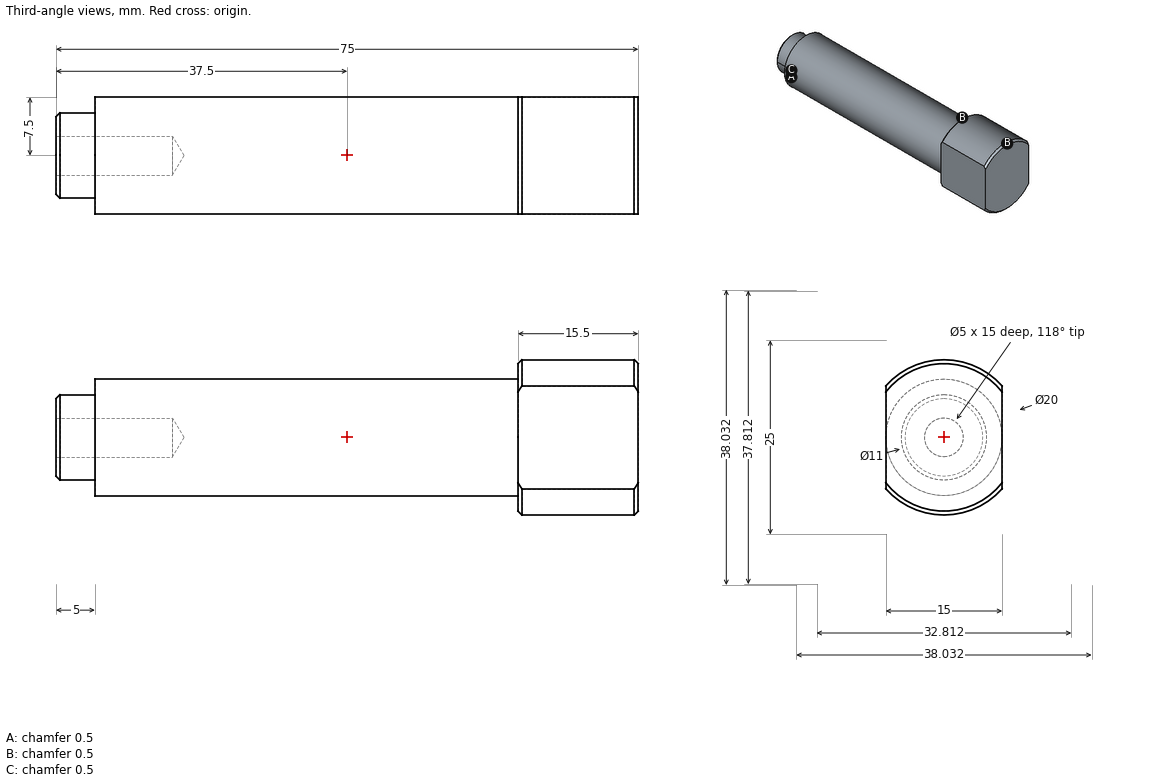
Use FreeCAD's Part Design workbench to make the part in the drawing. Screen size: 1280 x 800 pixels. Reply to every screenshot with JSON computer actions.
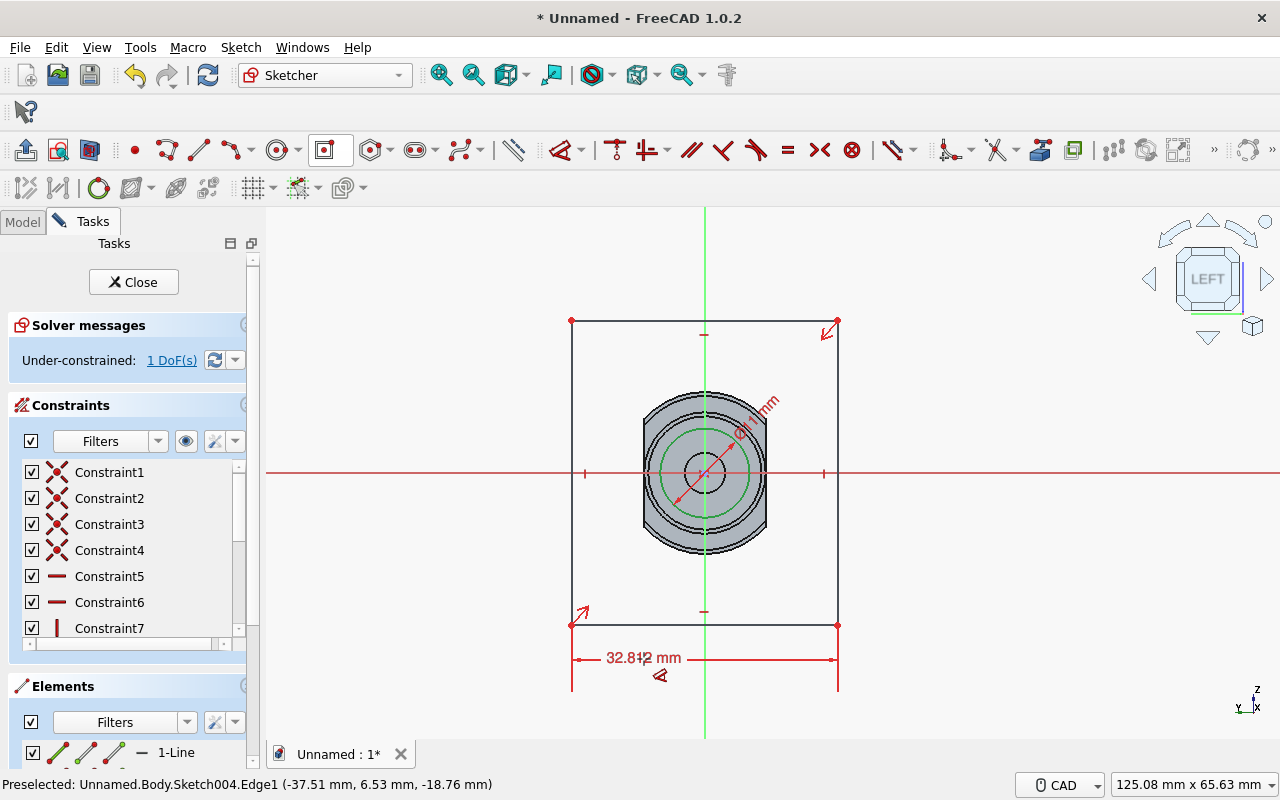
{"action": "left_click", "coordinate": [838, 534]}
{"action": "left_click", "coordinate": [872, 403]}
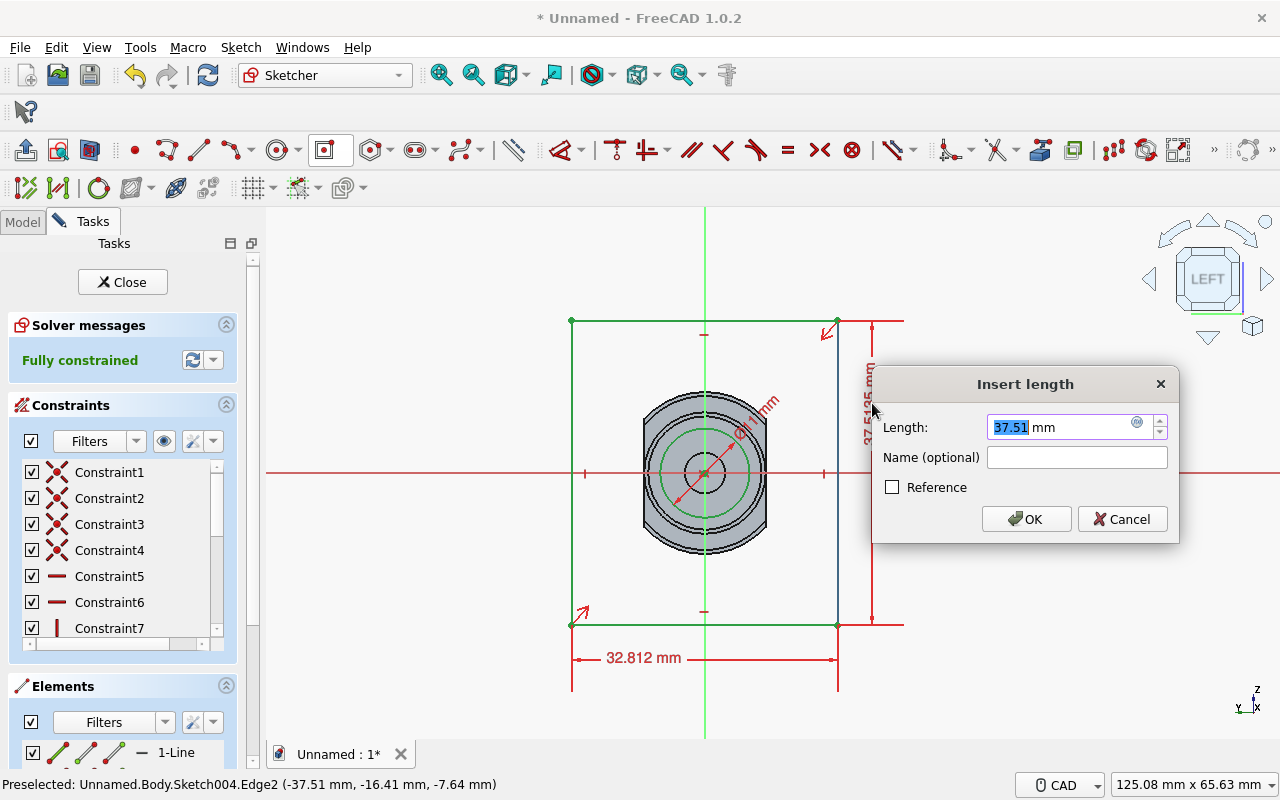
{"action": "type", "text": "37.812"}
{"action": "key", "text": "Return"}
{"action": "key", "text": "Escape"}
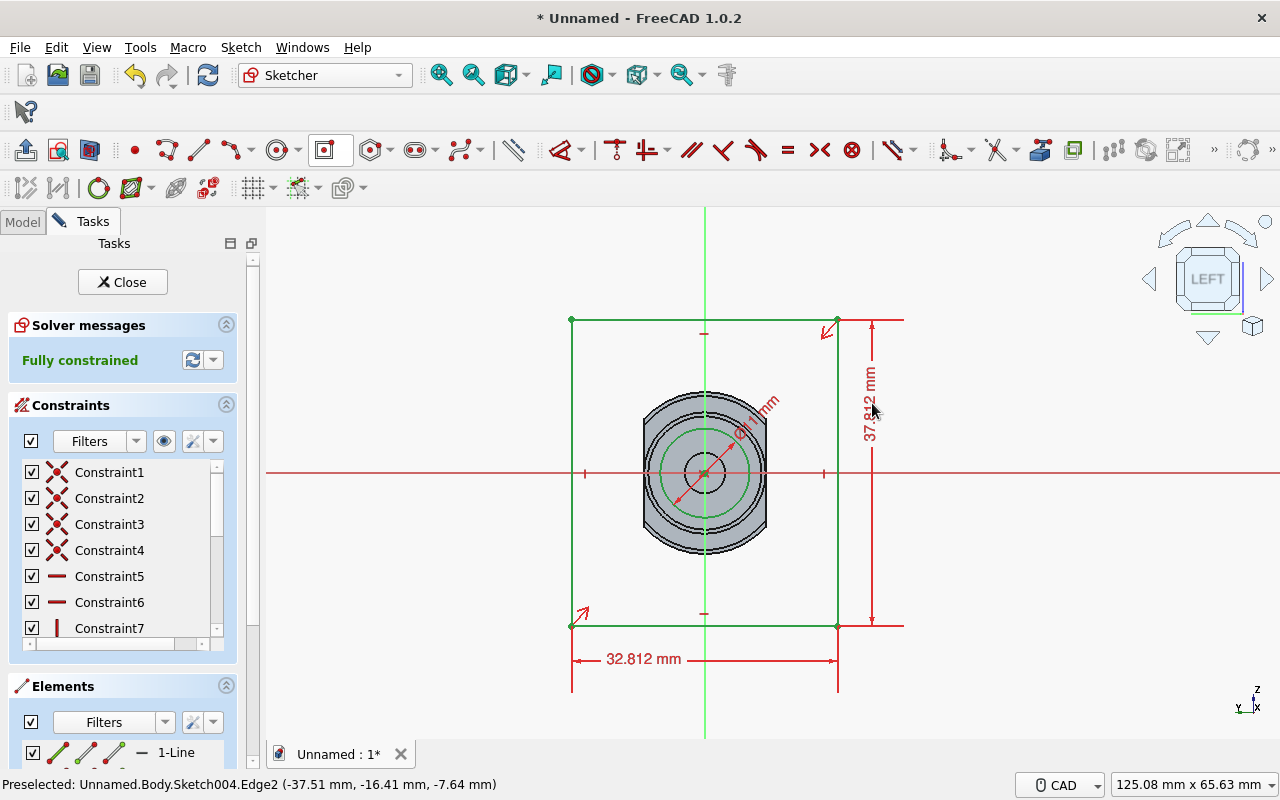
{"action": "left_click", "coordinate": [123, 282]}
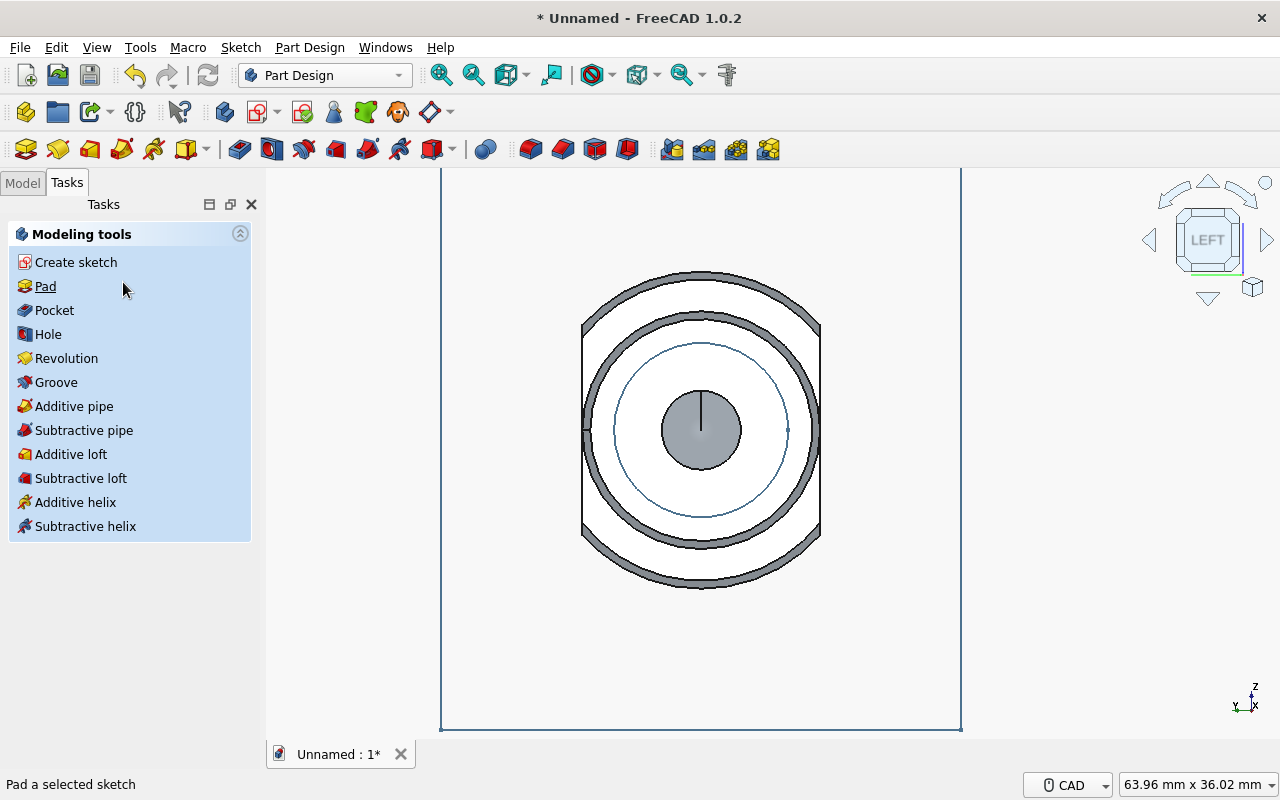
{"action": "left_click", "coordinate": [240, 150]}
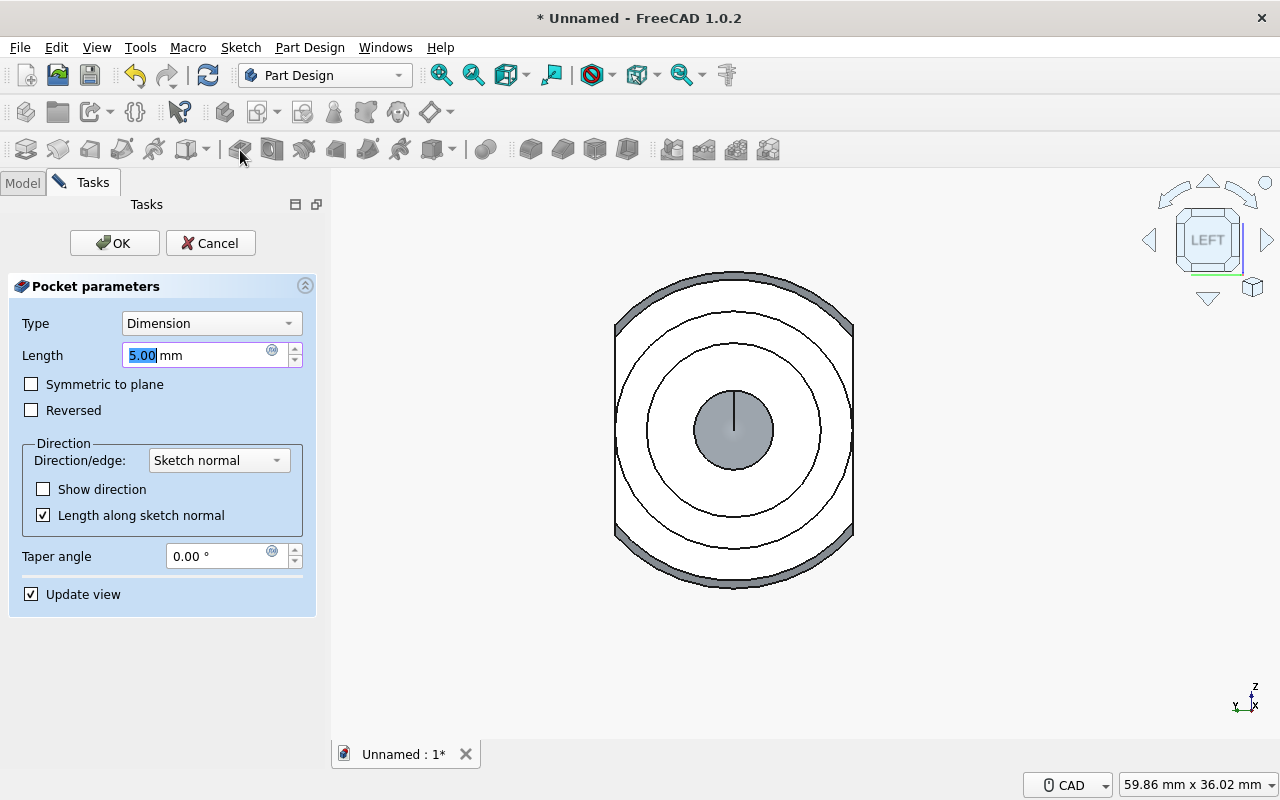
{"action": "type", "text": "5"}
{"action": "key", "text": "Tab"}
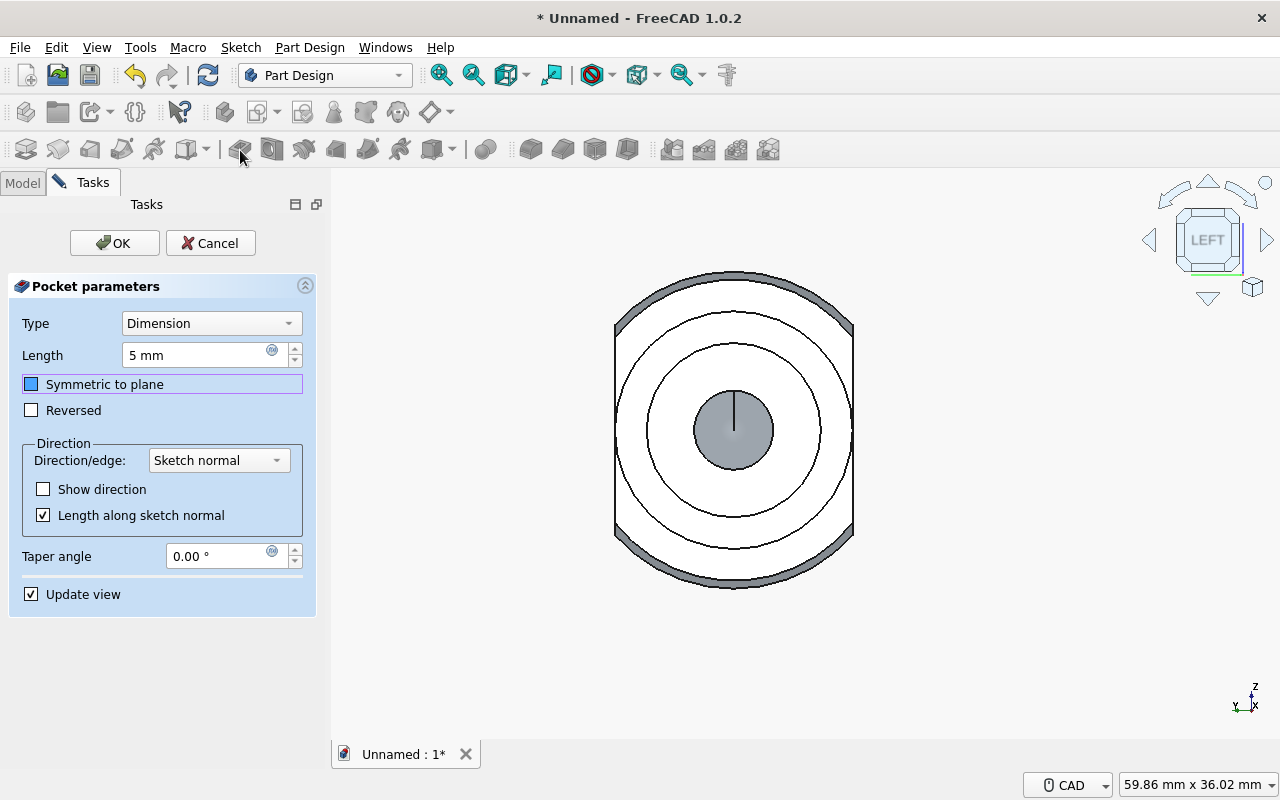
{"action": "left_click", "coordinate": [115, 243]}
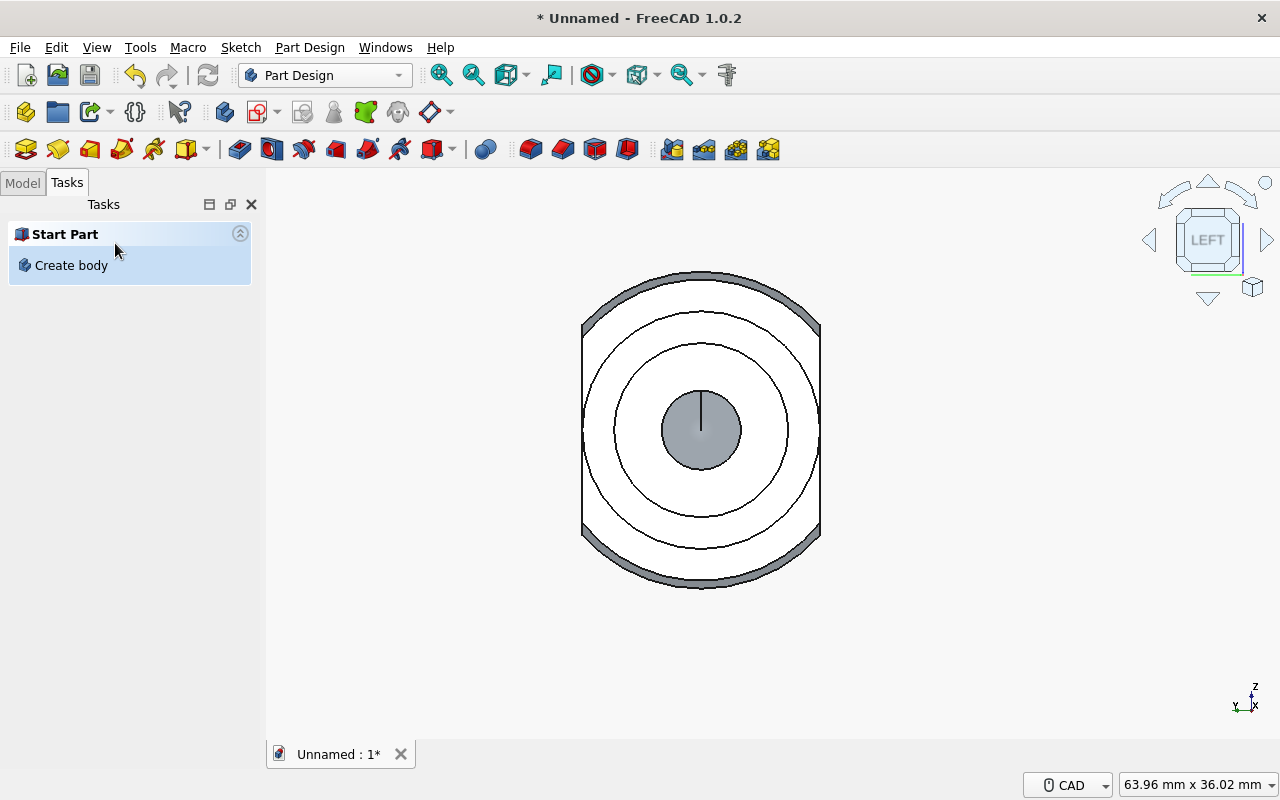
{"action": "left_click", "coordinate": [614, 429]}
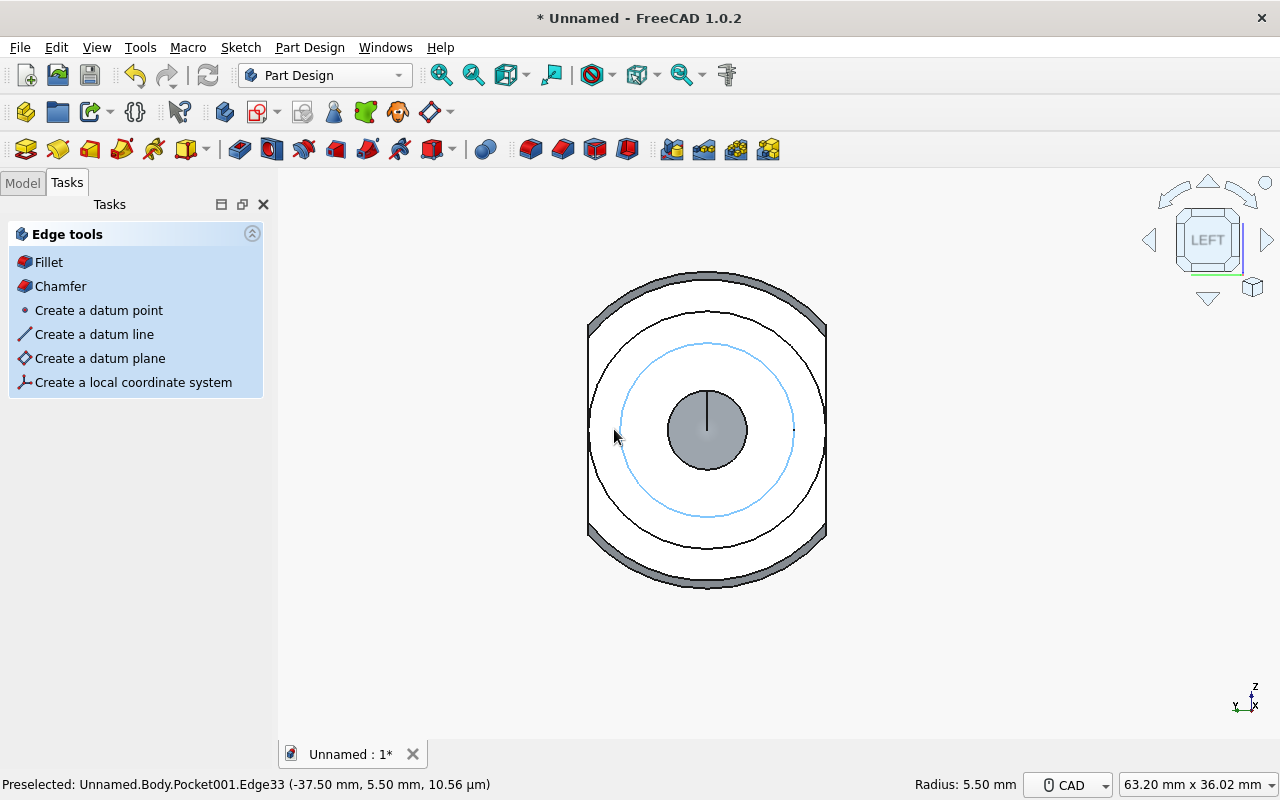
{"action": "left_click", "coordinate": [564, 150]}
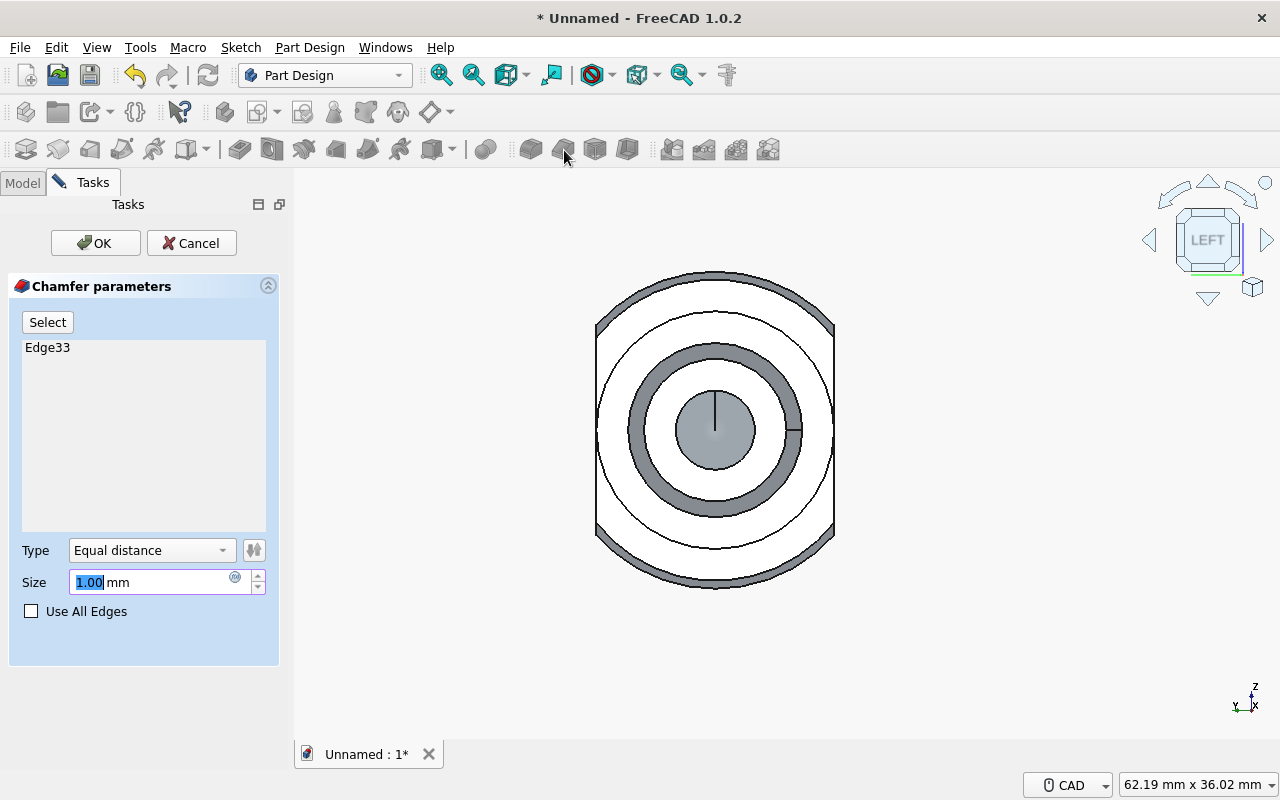
{"action": "type", "text": "0.5"}
{"action": "key", "text": "Tab"}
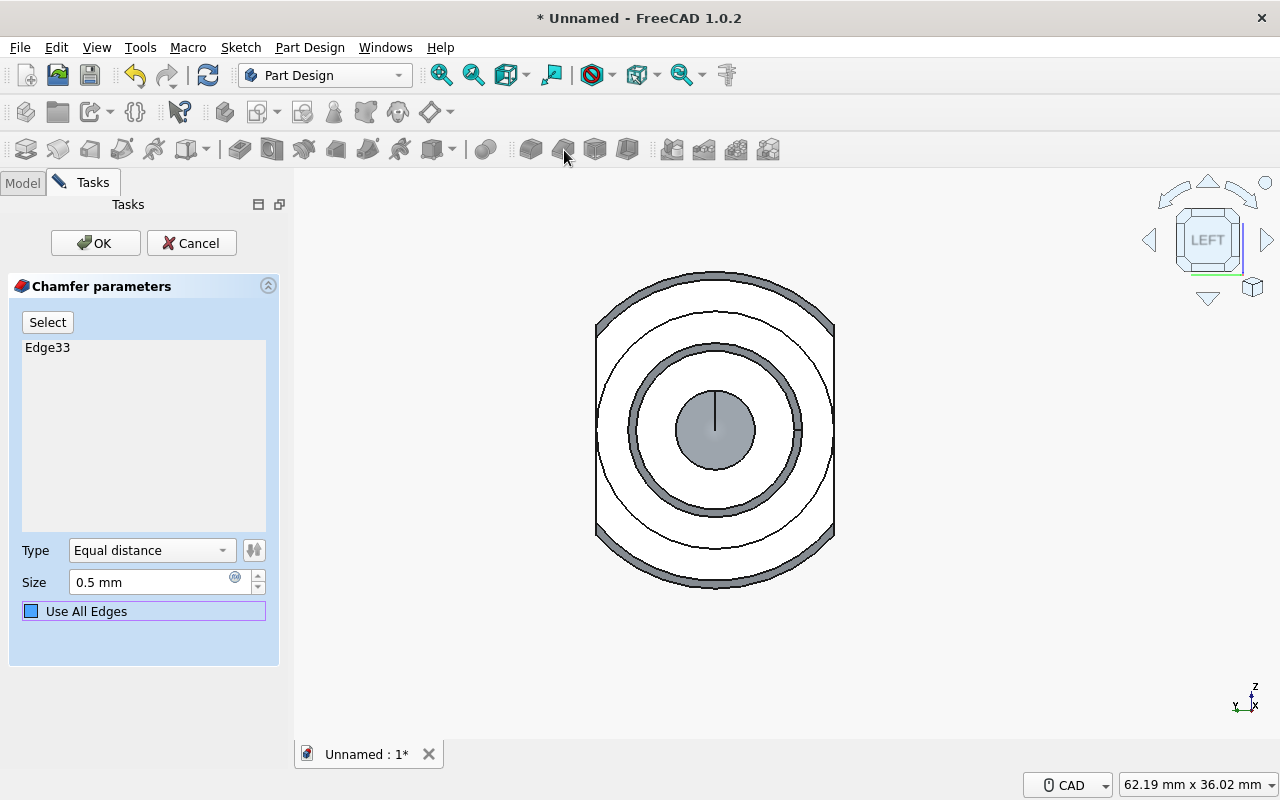
{"action": "left_click", "coordinate": [96, 243]}